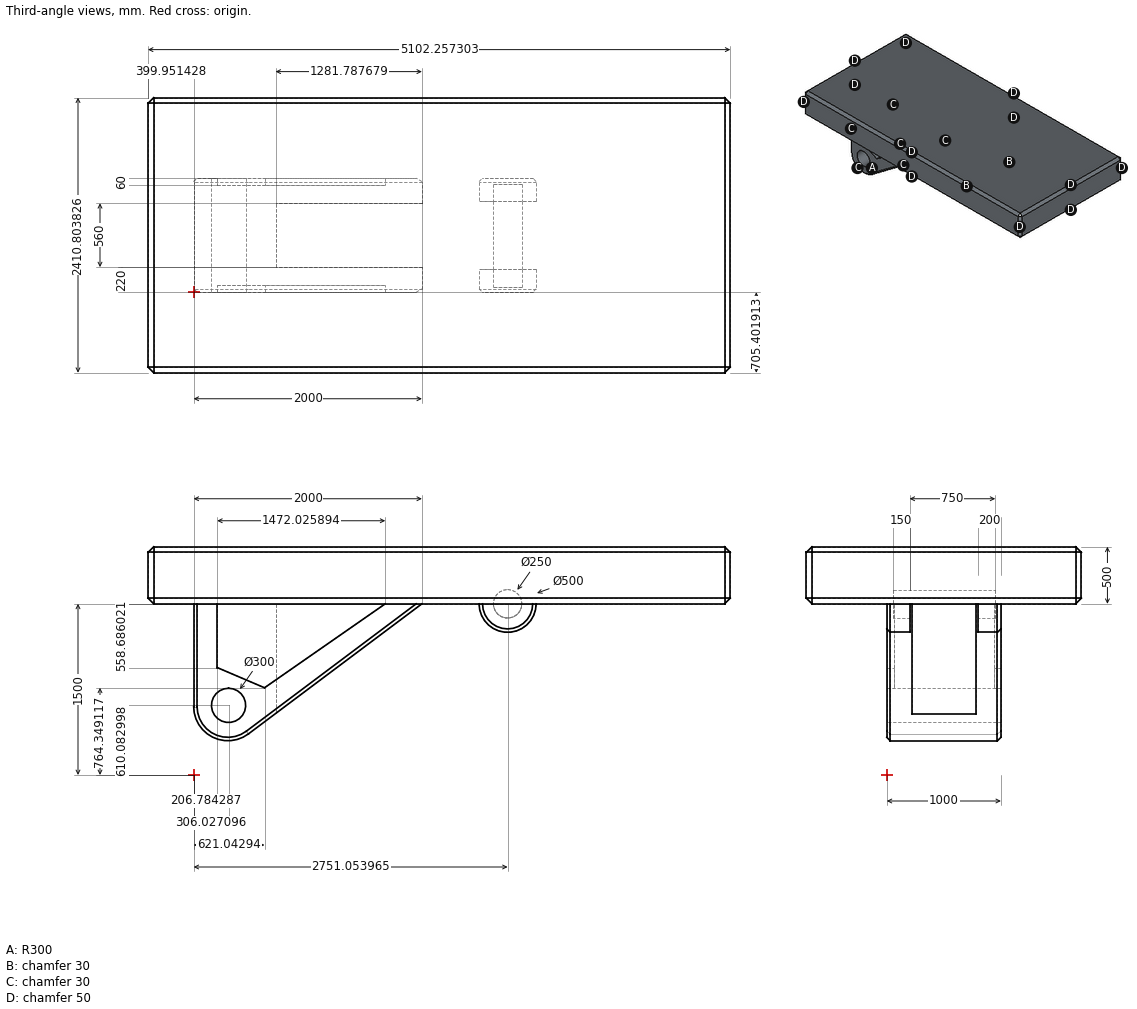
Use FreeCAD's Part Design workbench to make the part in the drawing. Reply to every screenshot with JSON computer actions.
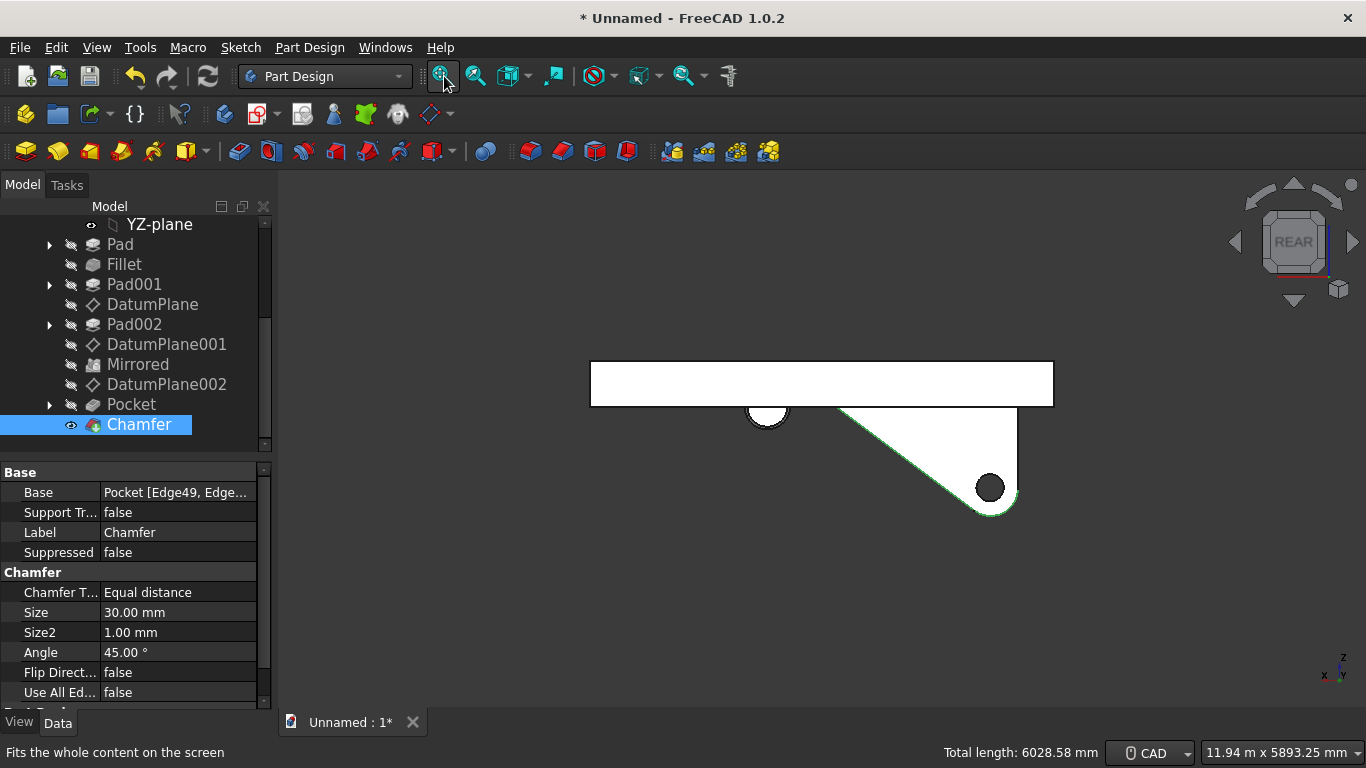
{"action": "left_click", "coordinate": [1018, 447], "text": "ctrl"}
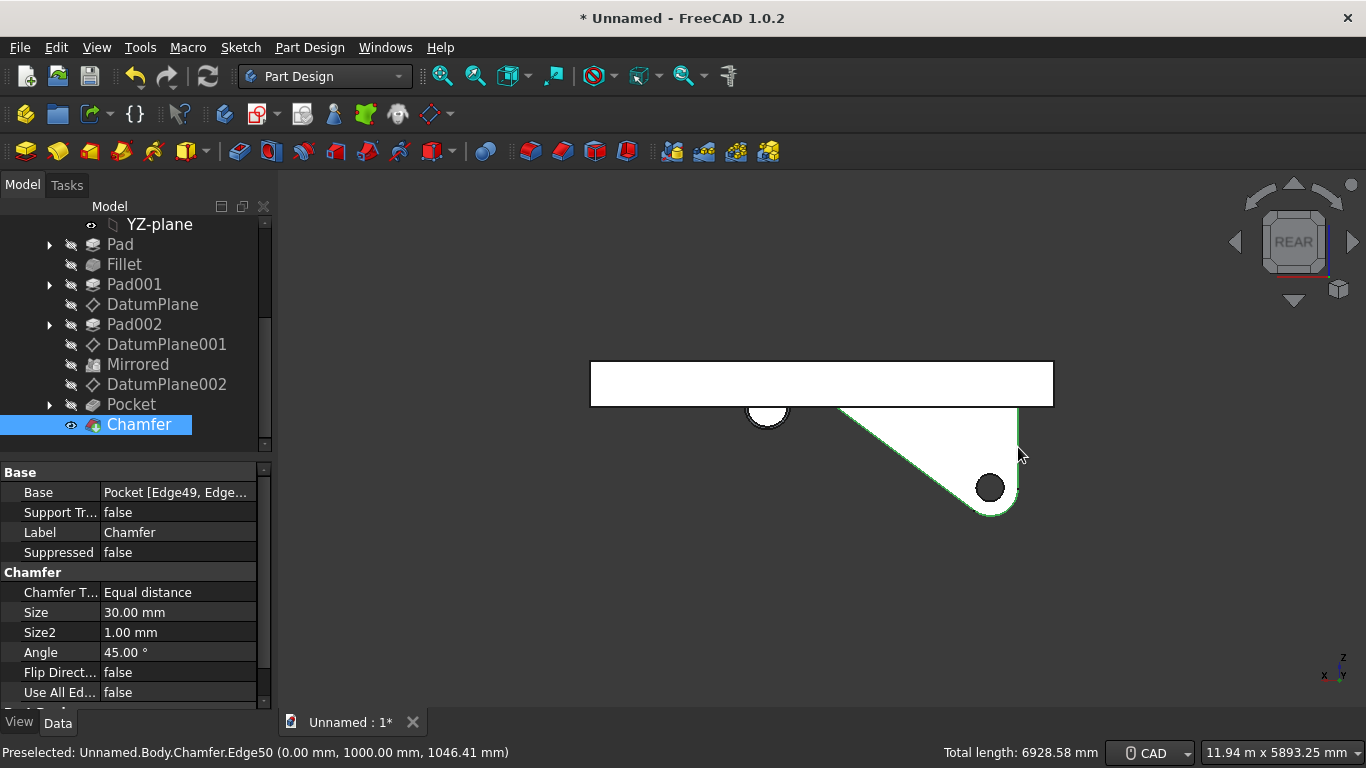
{"action": "left_click", "coordinate": [564, 152]}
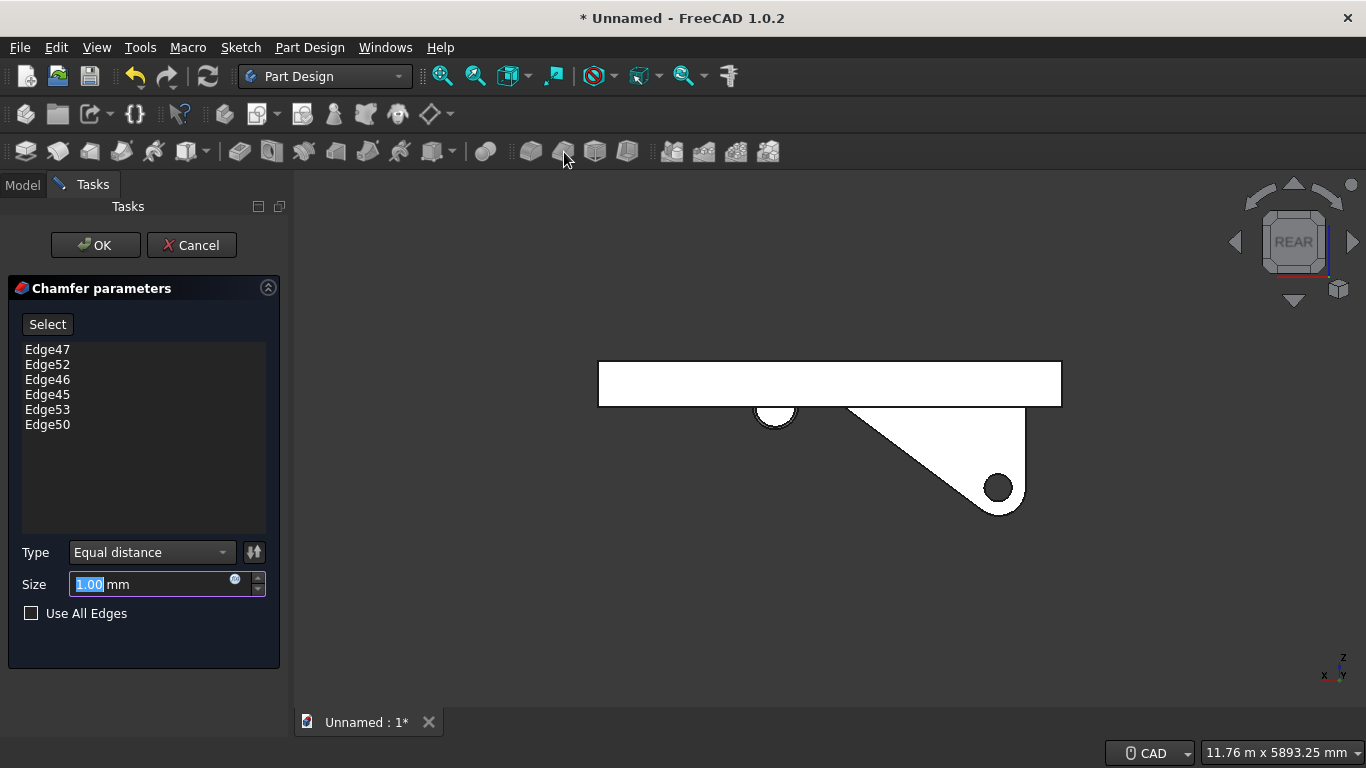
{"action": "type", "text": "30"}
{"action": "key", "text": "Tab"}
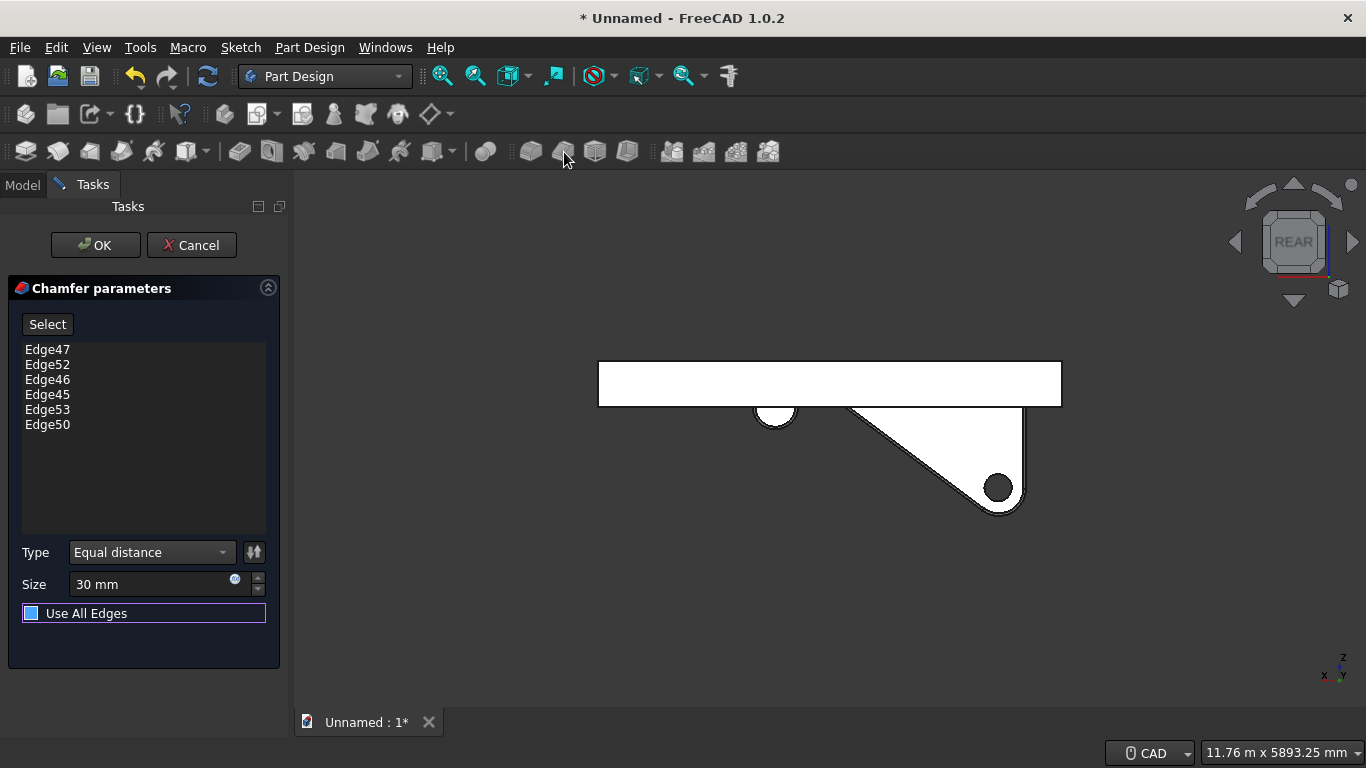
{"action": "left_click", "coordinate": [96, 245]}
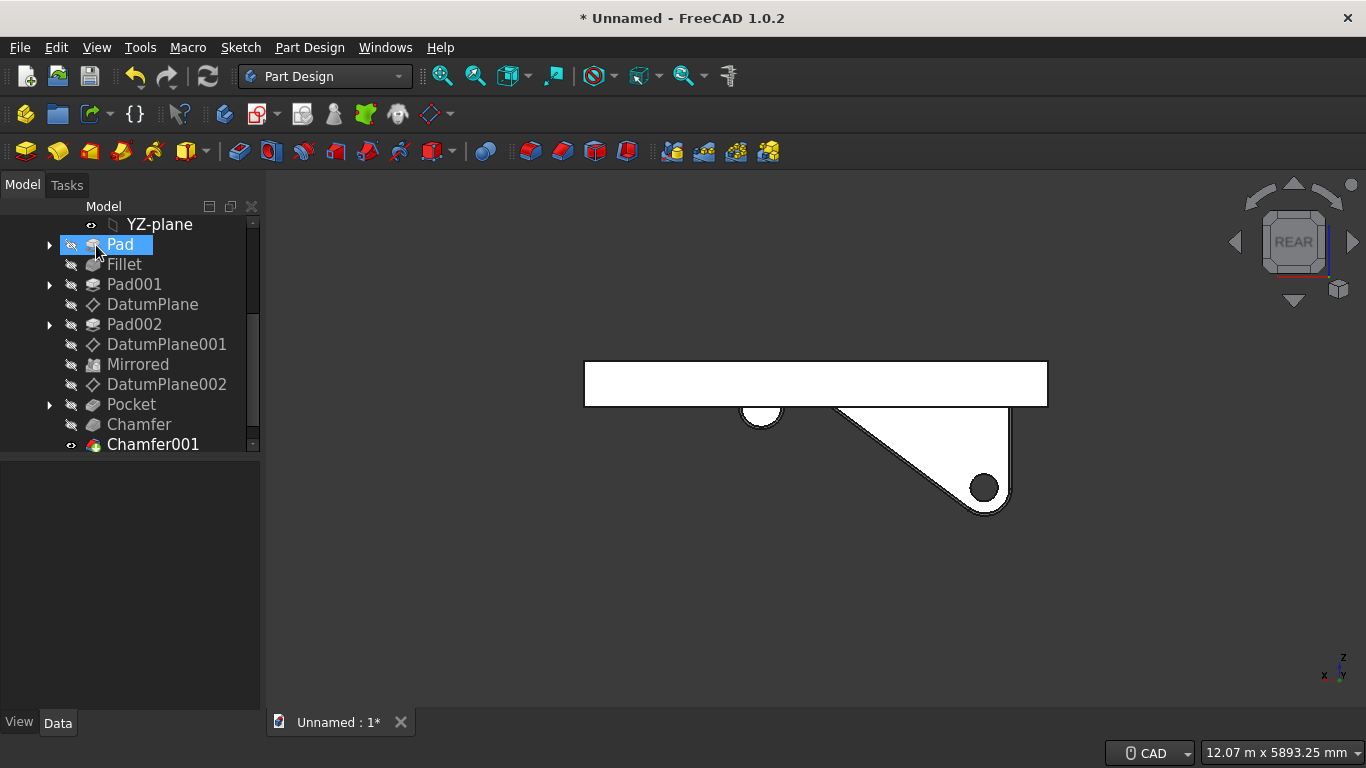
{"action": "left_click", "coordinate": [444, 76]}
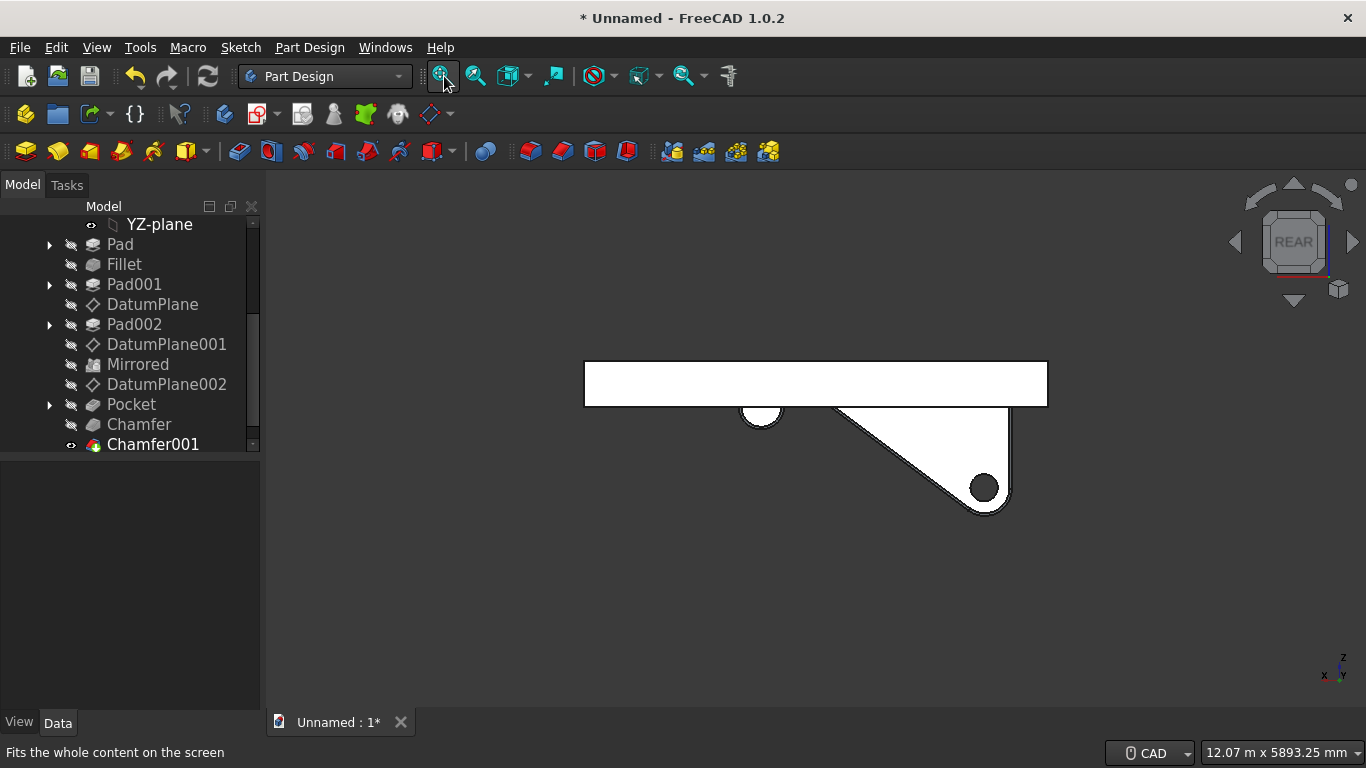
{"action": "left_click", "coordinate": [947, 444]}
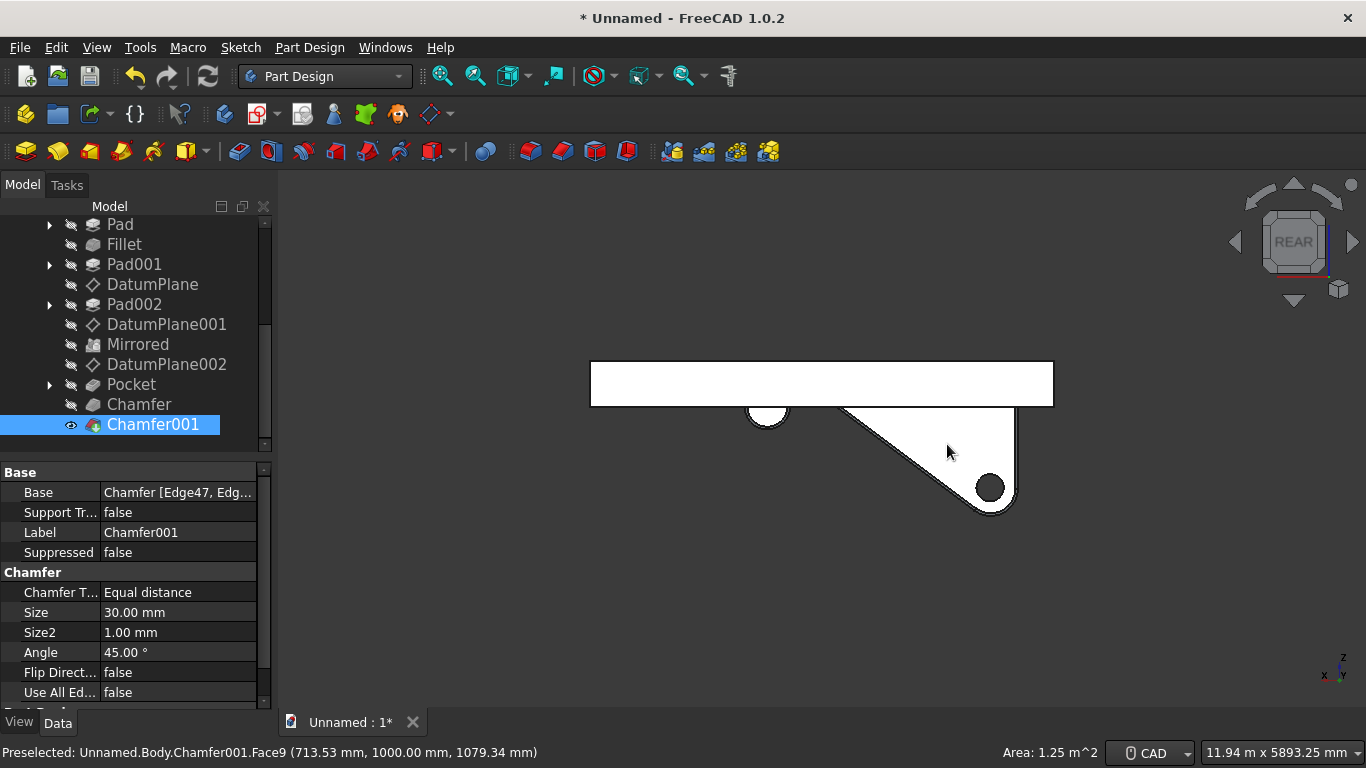
{"action": "left_click", "coordinate": [258, 114]}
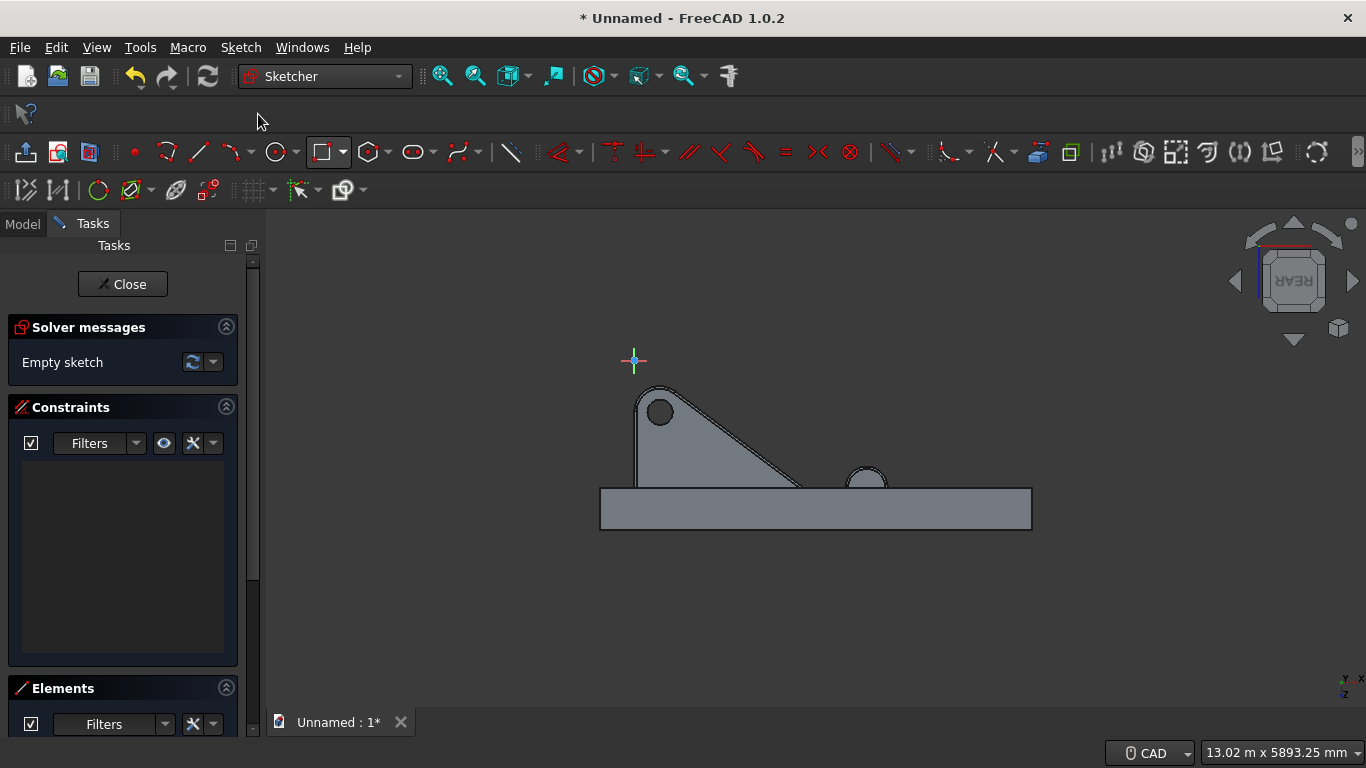
{"action": "left_click", "coordinate": [90, 152]}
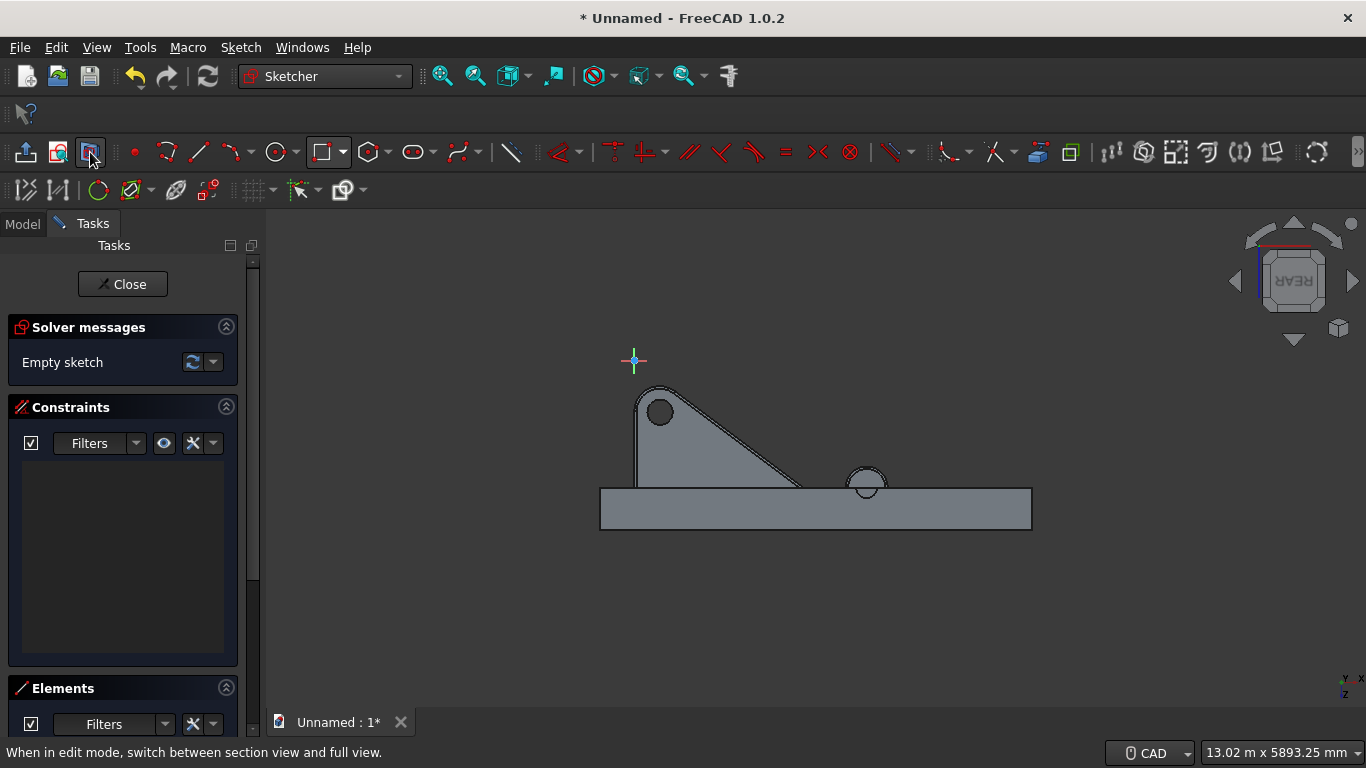
{"action": "scroll", "coordinate": [681, 404], "scroll_direction": "up", "scroll_amount": 5}